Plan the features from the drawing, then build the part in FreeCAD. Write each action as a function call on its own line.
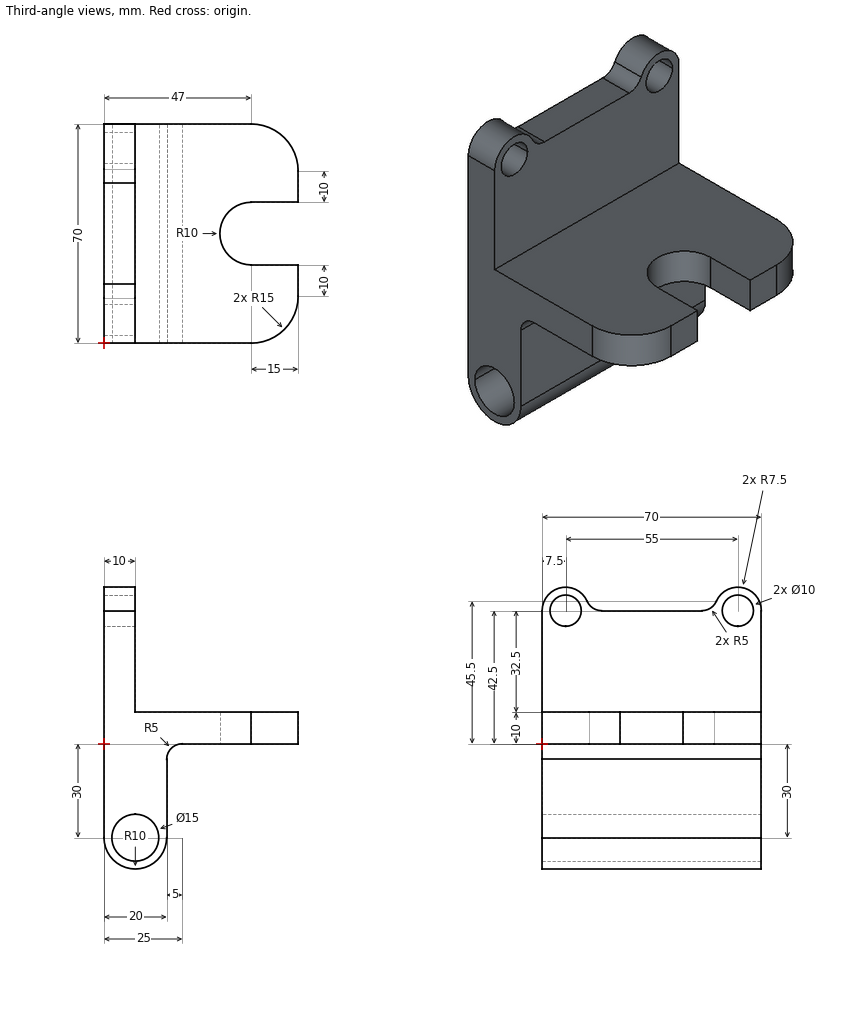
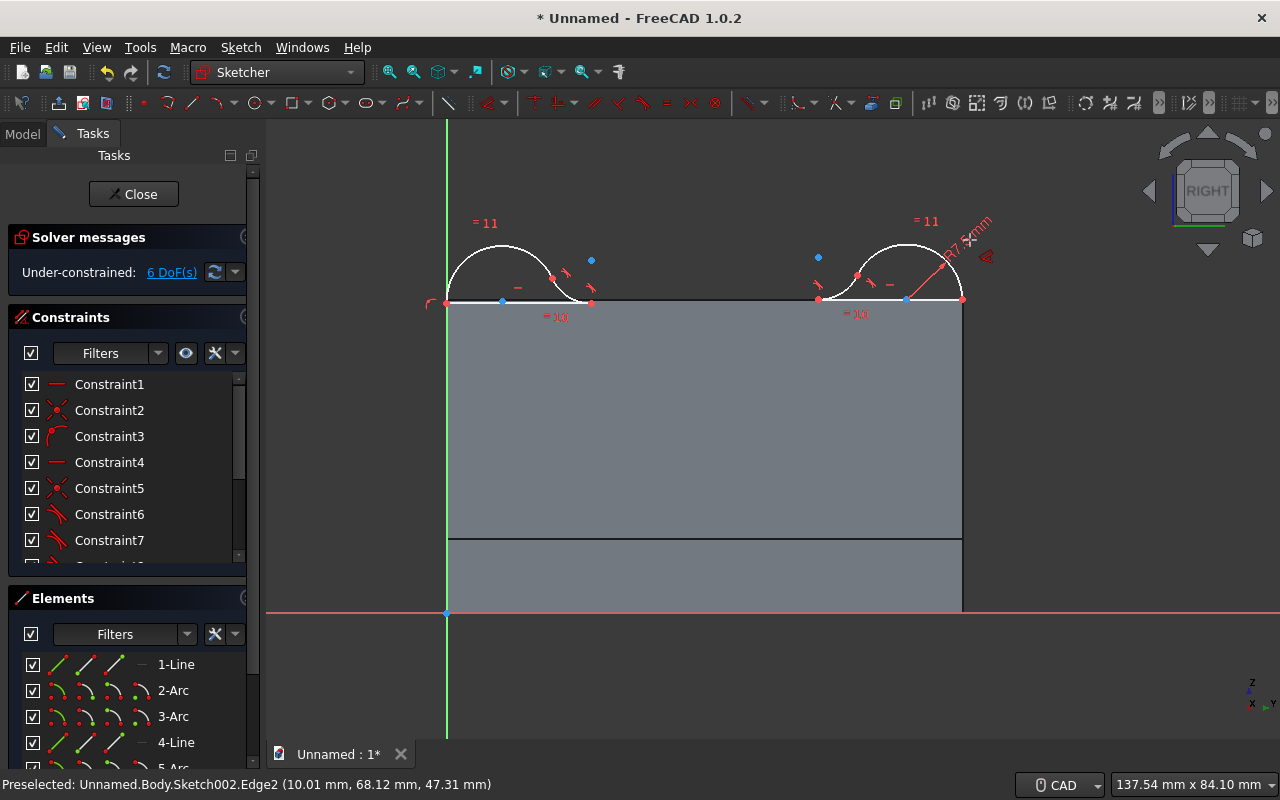
click(849, 287)
click(840, 328)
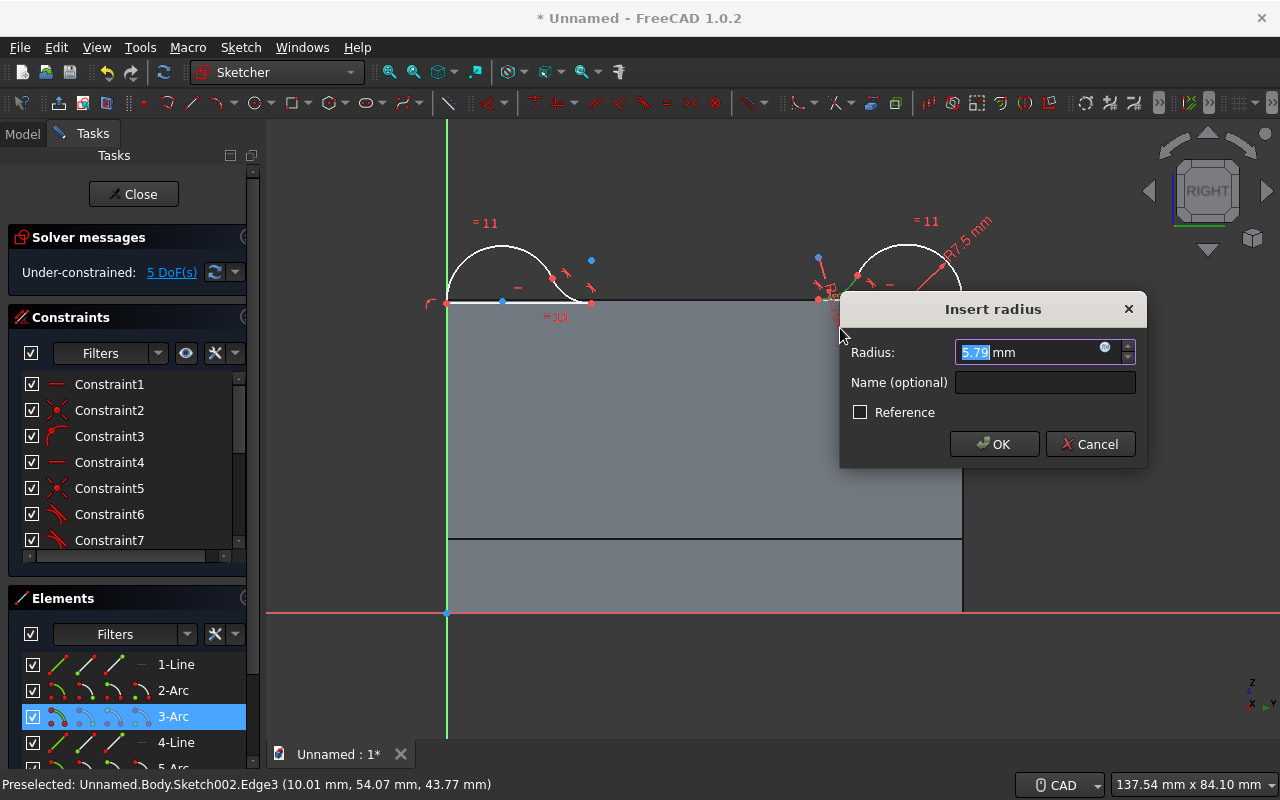
text(5)
key(Return)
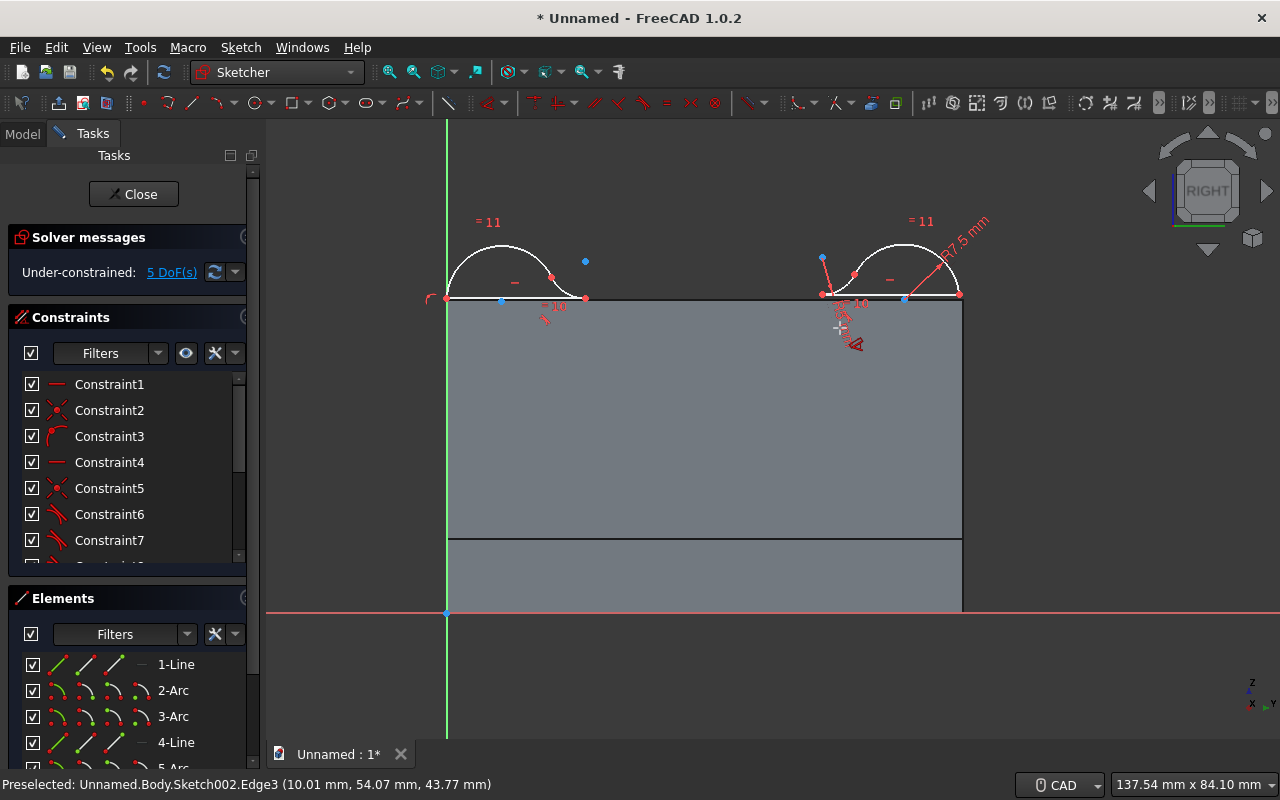
click(959, 295)
click(703, 647)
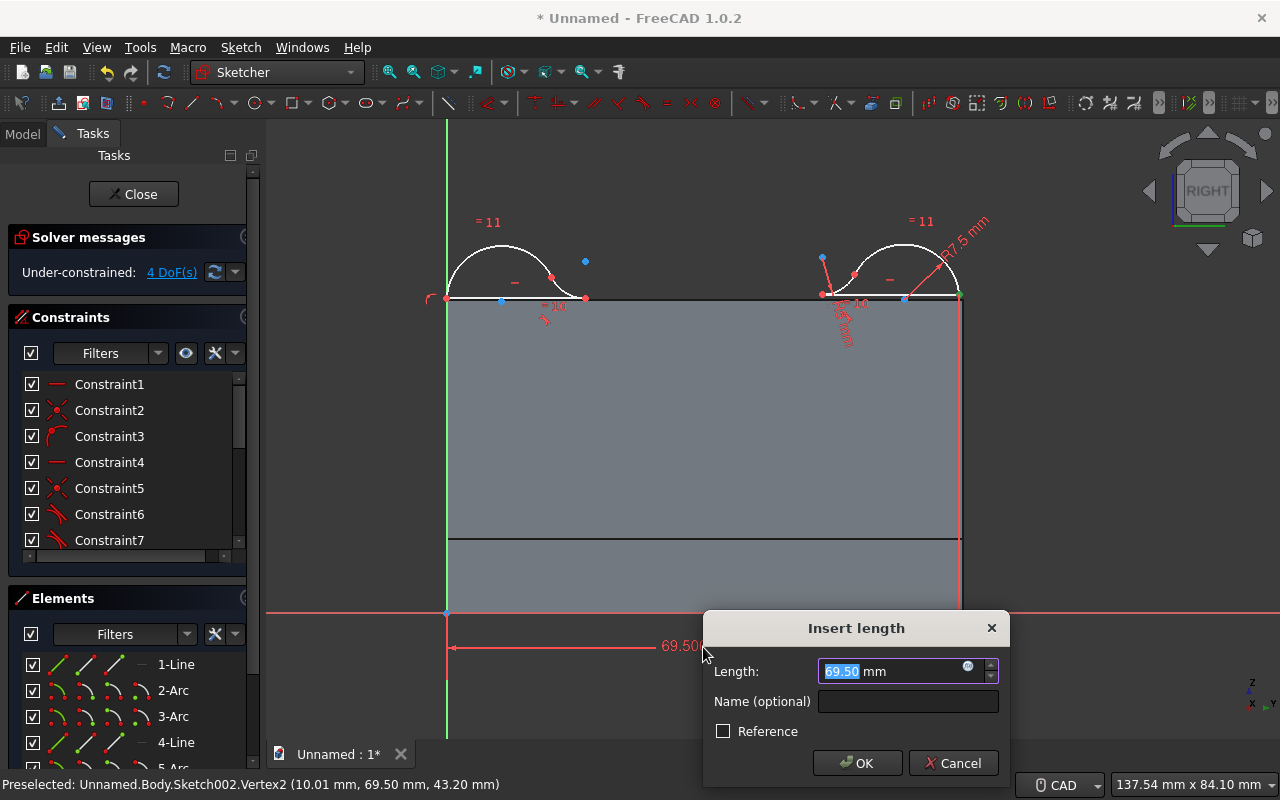
text(70)
key(Return)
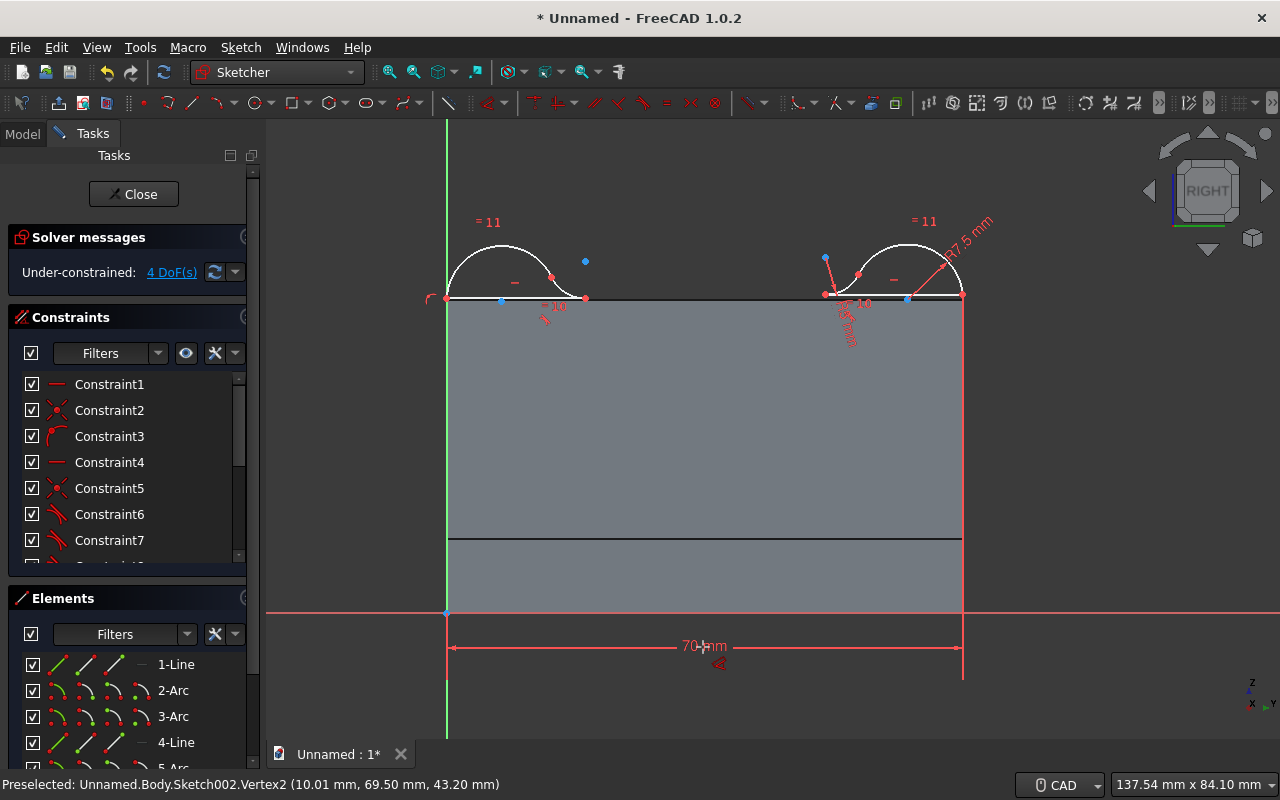
click(826, 295)
click(413, 454)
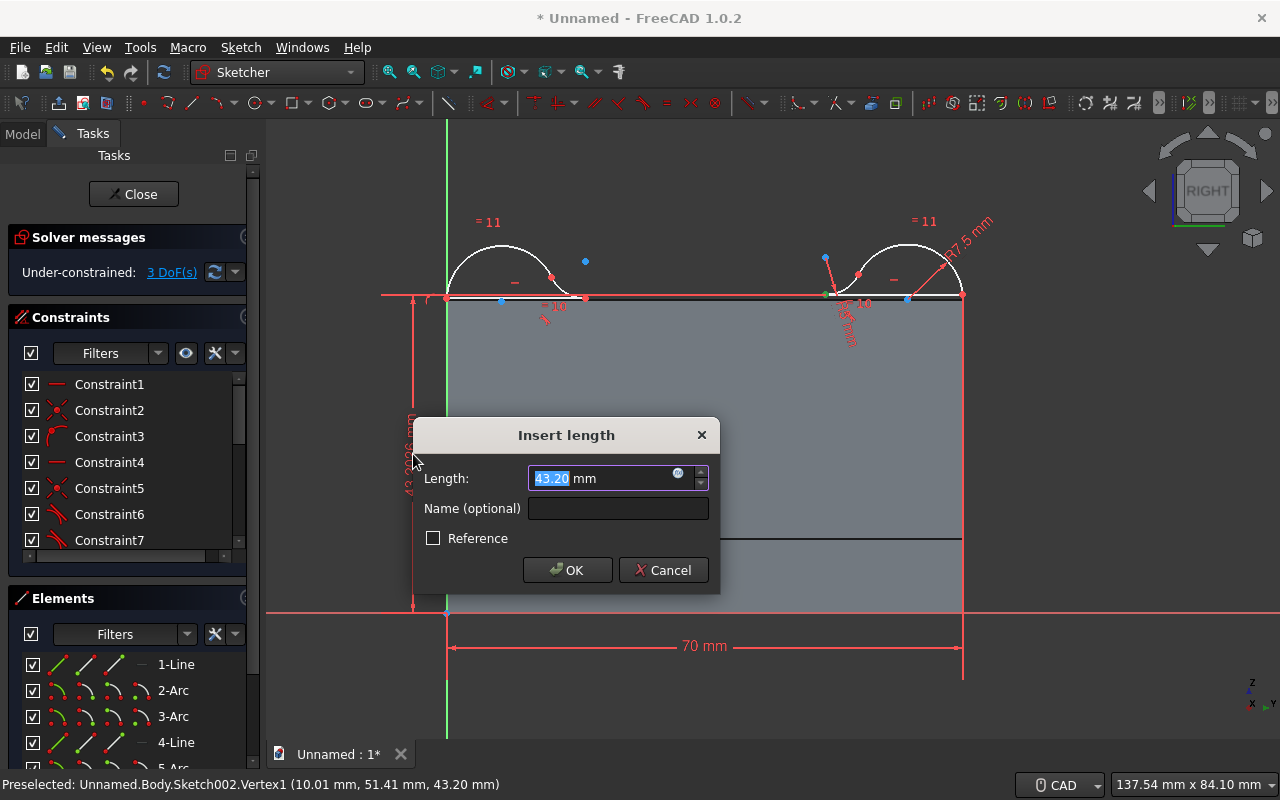
text(42.5)
key(Return)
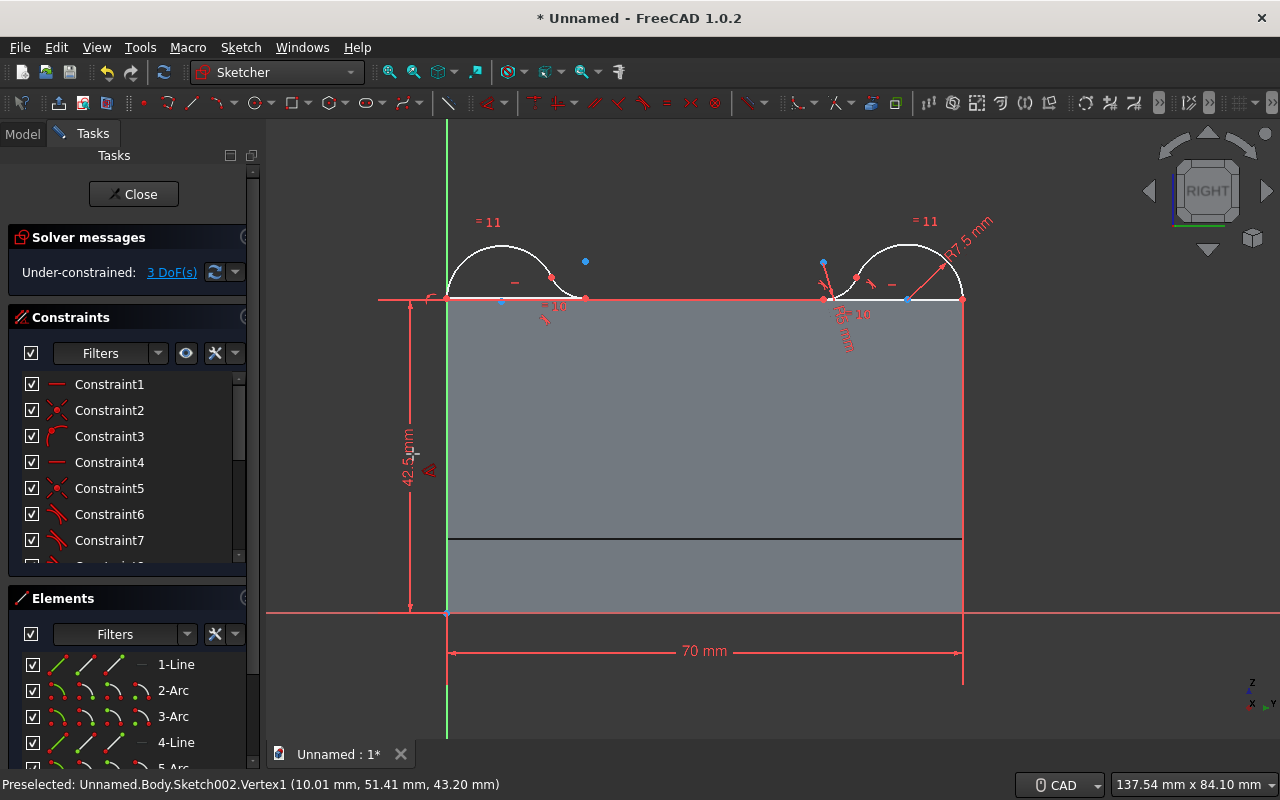
click(857, 278)
click(413, 368)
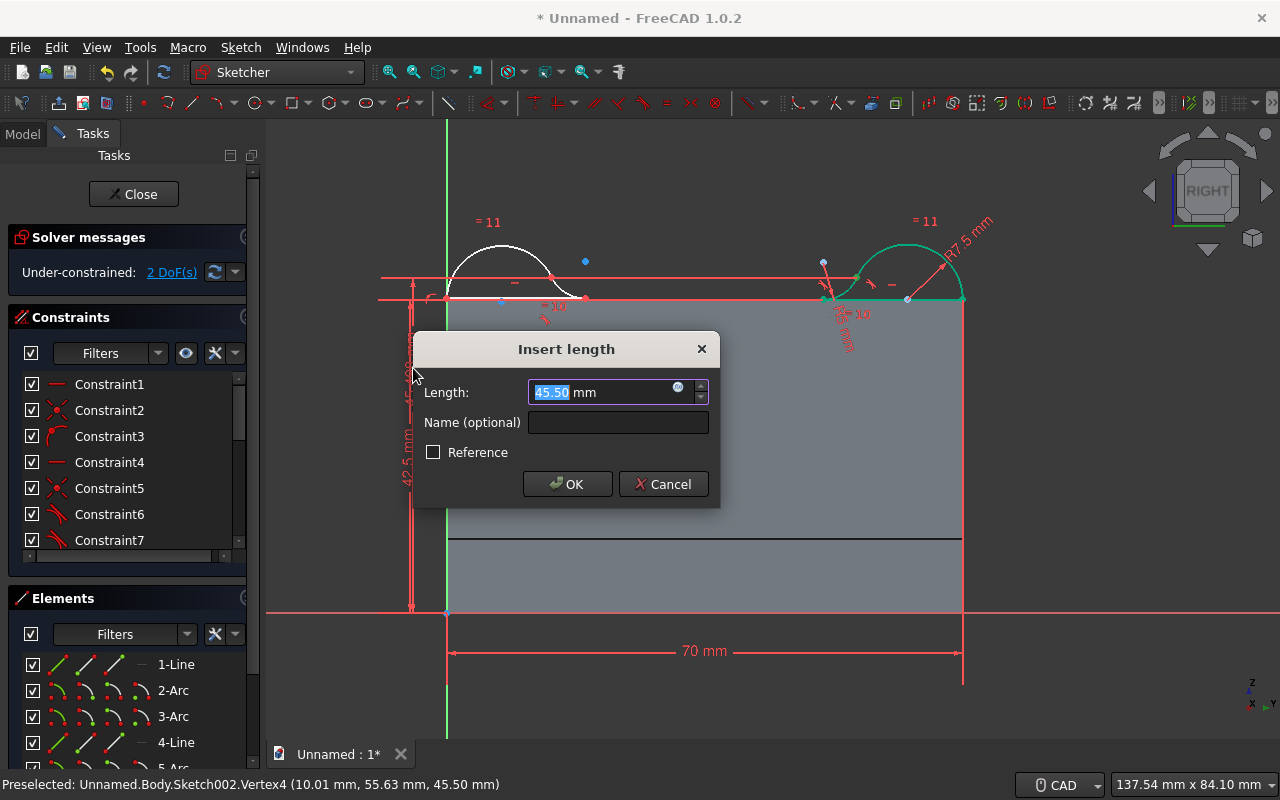
text(45.5)
key(Return)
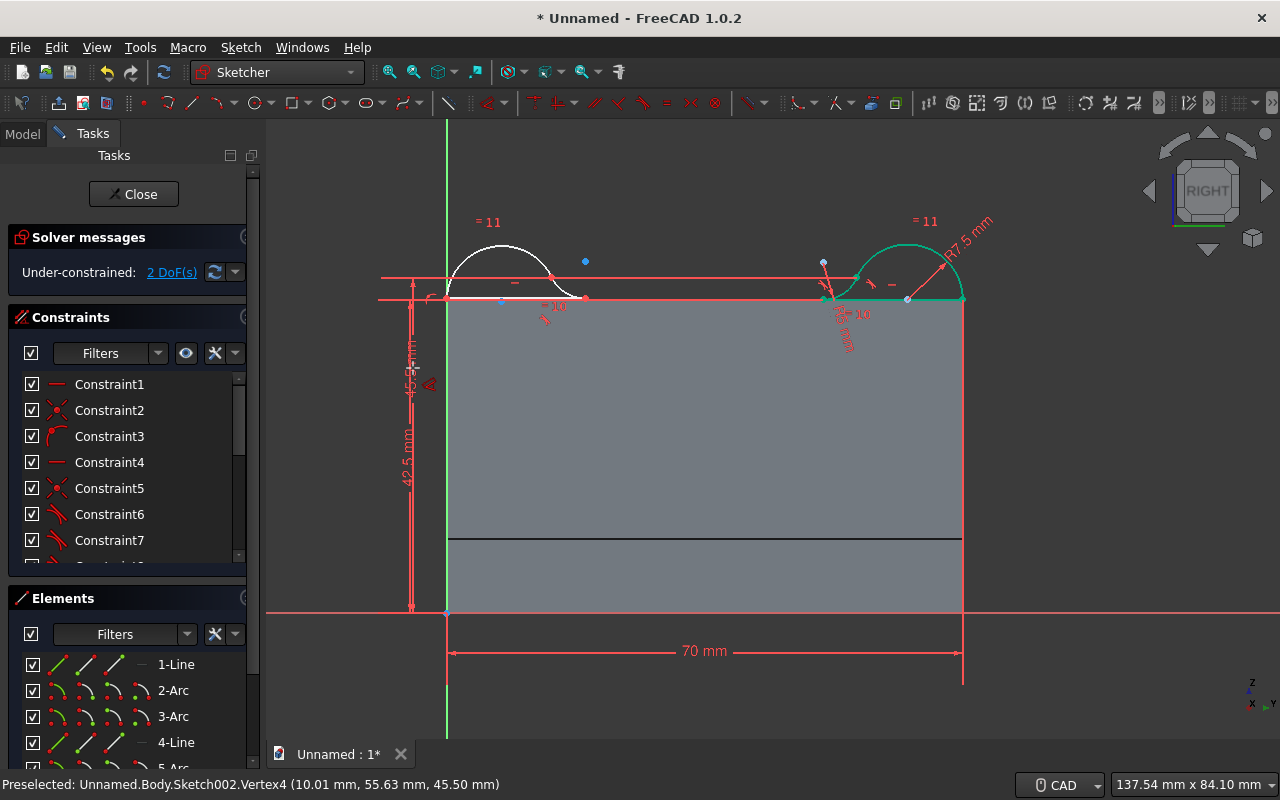
click(447, 298)
click(413, 528)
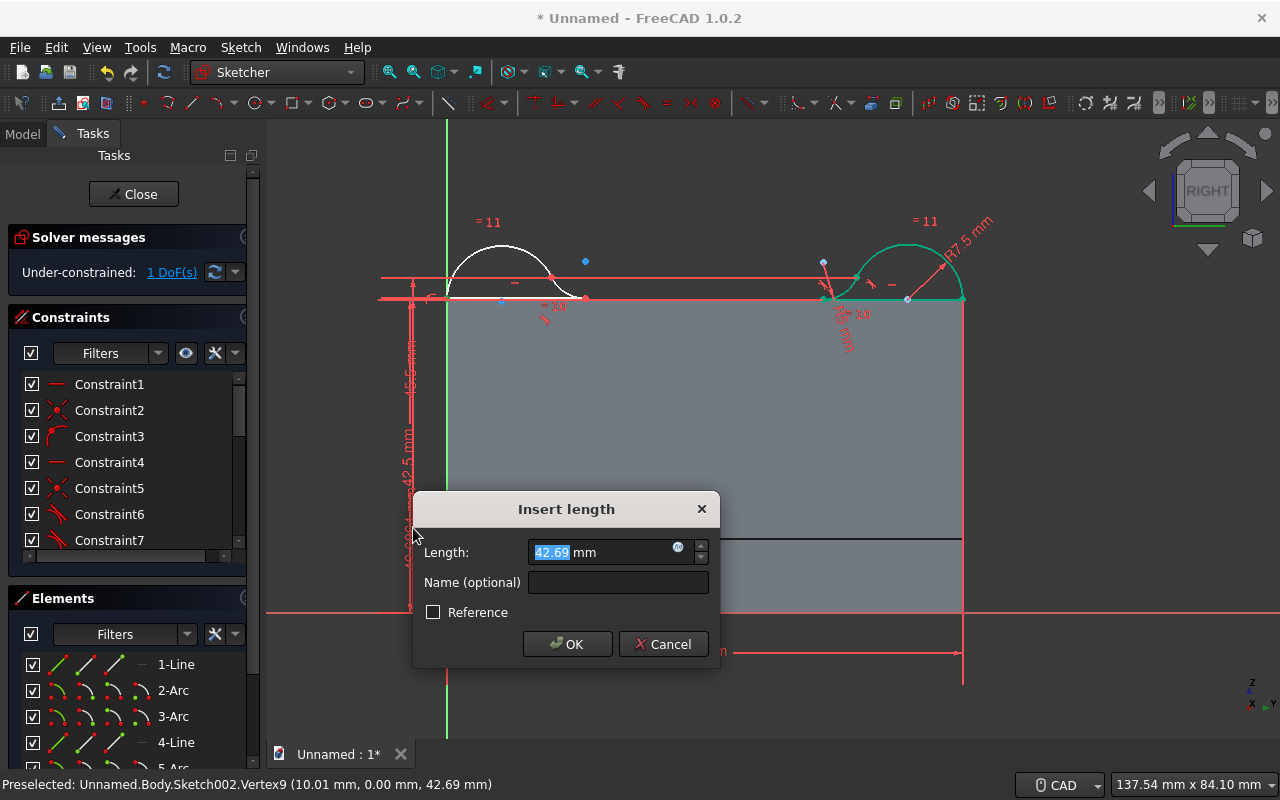
text(42.5)
key(Return)